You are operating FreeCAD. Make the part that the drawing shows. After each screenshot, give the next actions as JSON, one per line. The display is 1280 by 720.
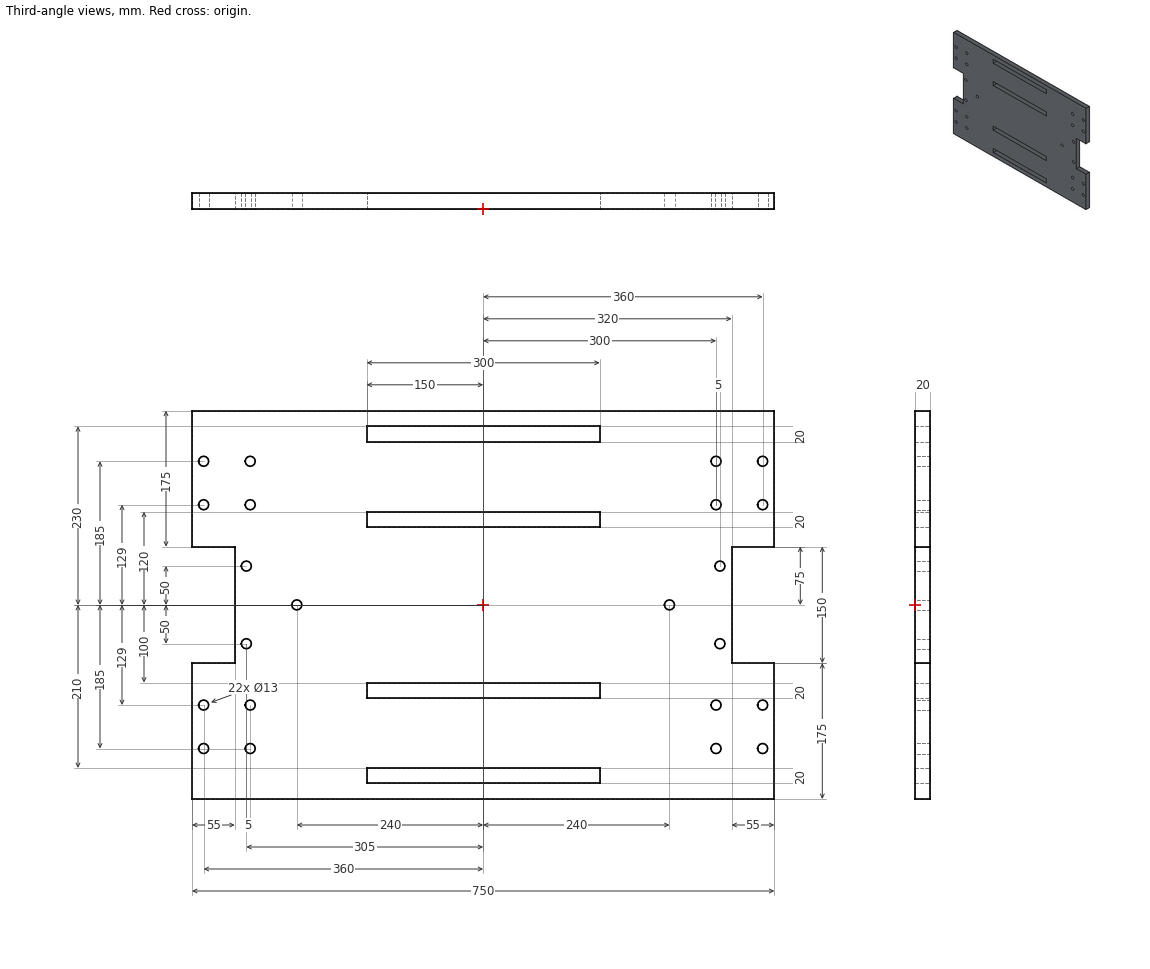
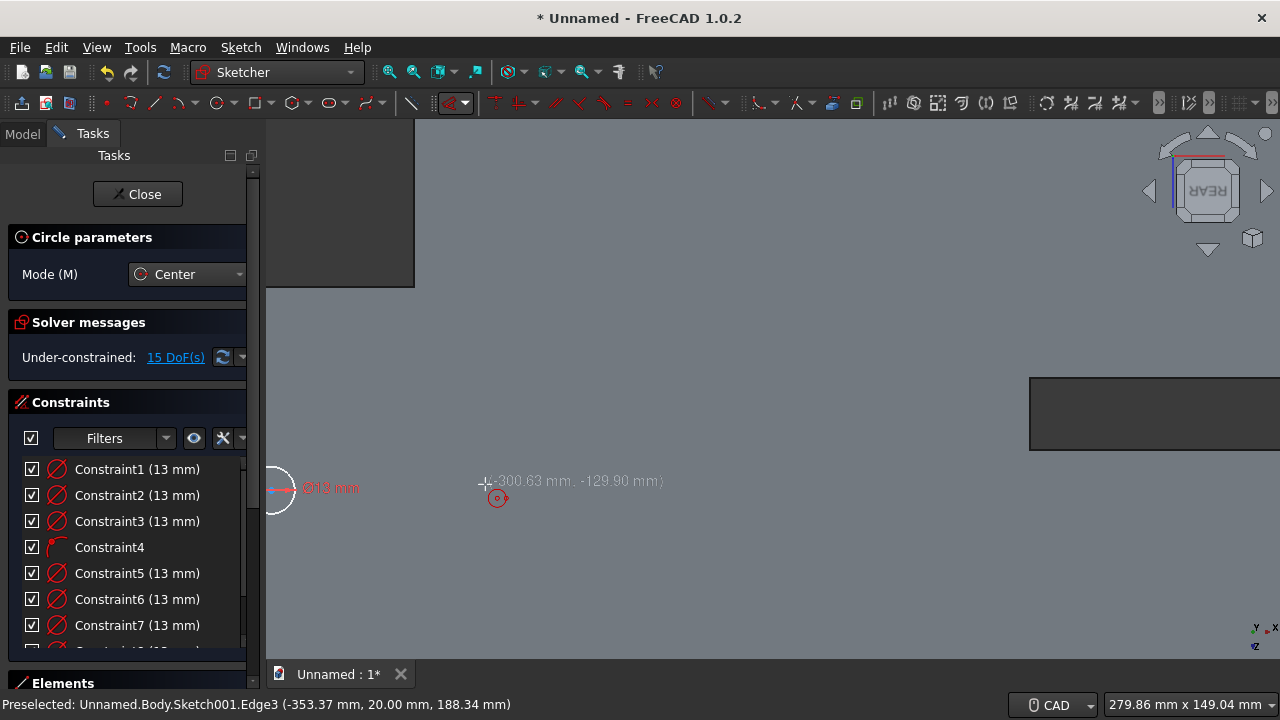
{"action": "scroll", "coordinate": [485, 483], "scroll_direction": "down", "scroll_amount": 8}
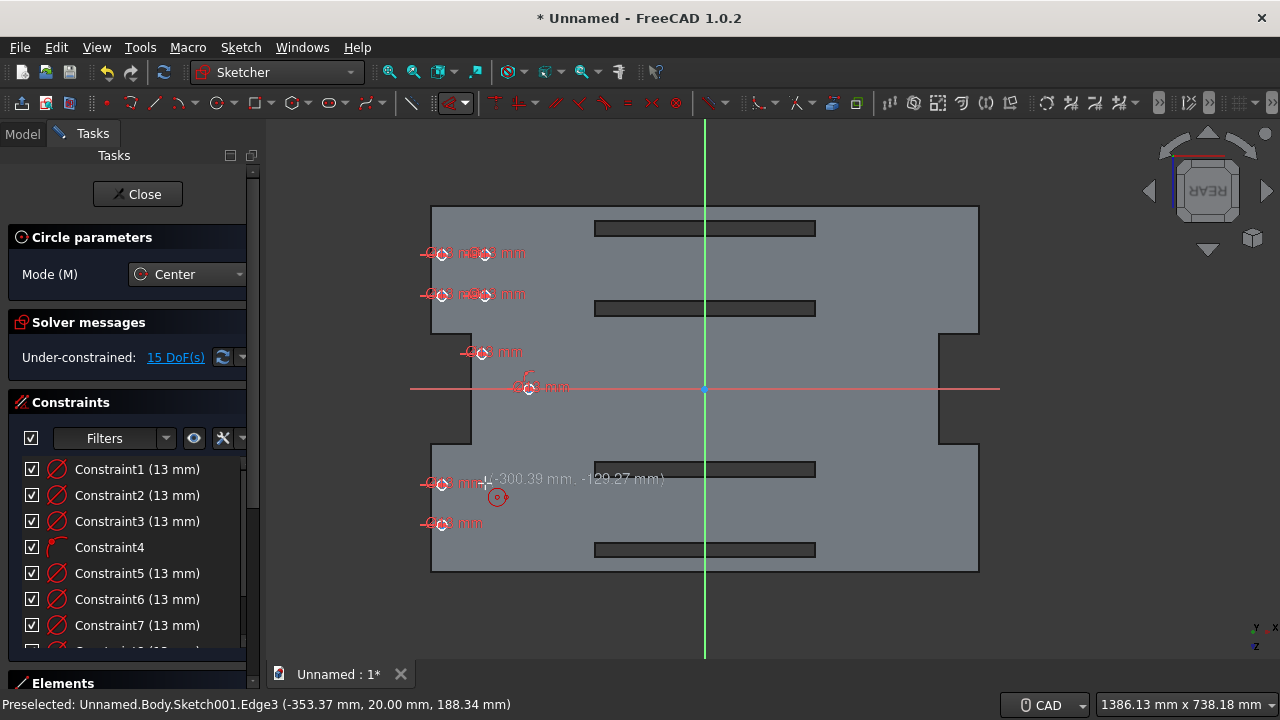
{"action": "left_click", "coordinate": [485, 484]}
{"action": "mouse_move", "coordinate": [489, 480]}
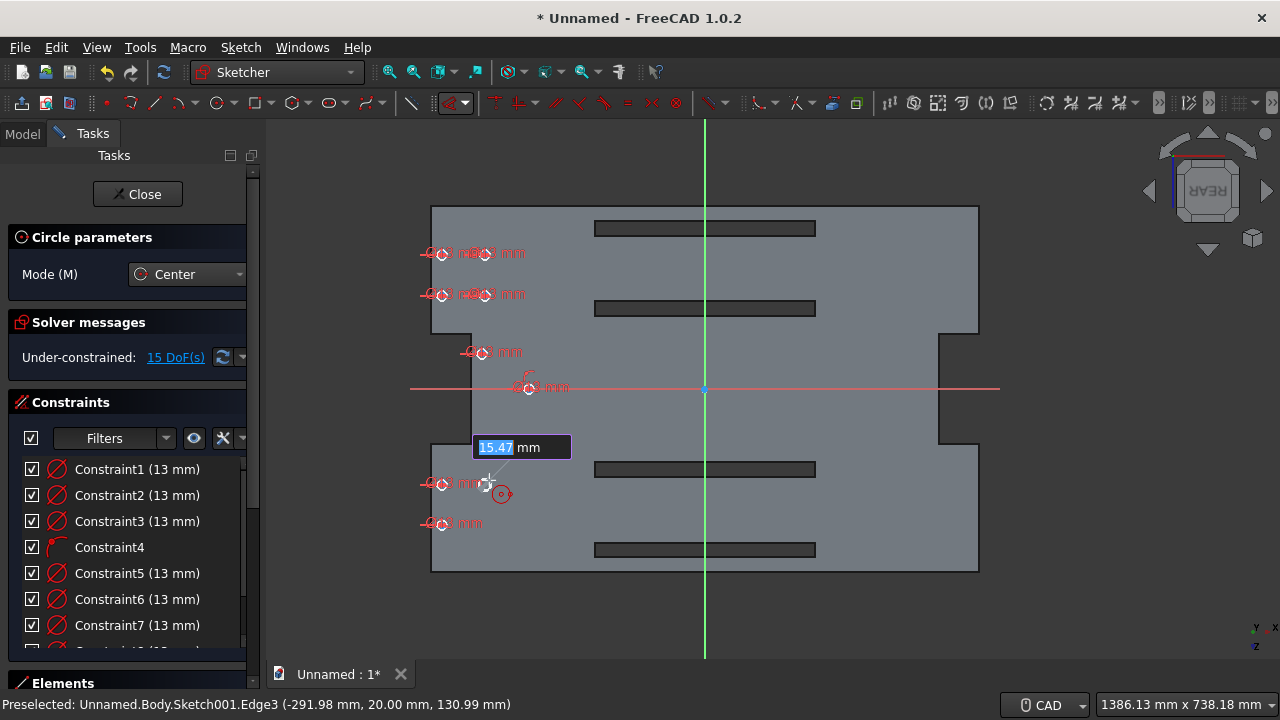
{"action": "type", "text": "13"}
{"action": "key", "text": "Return"}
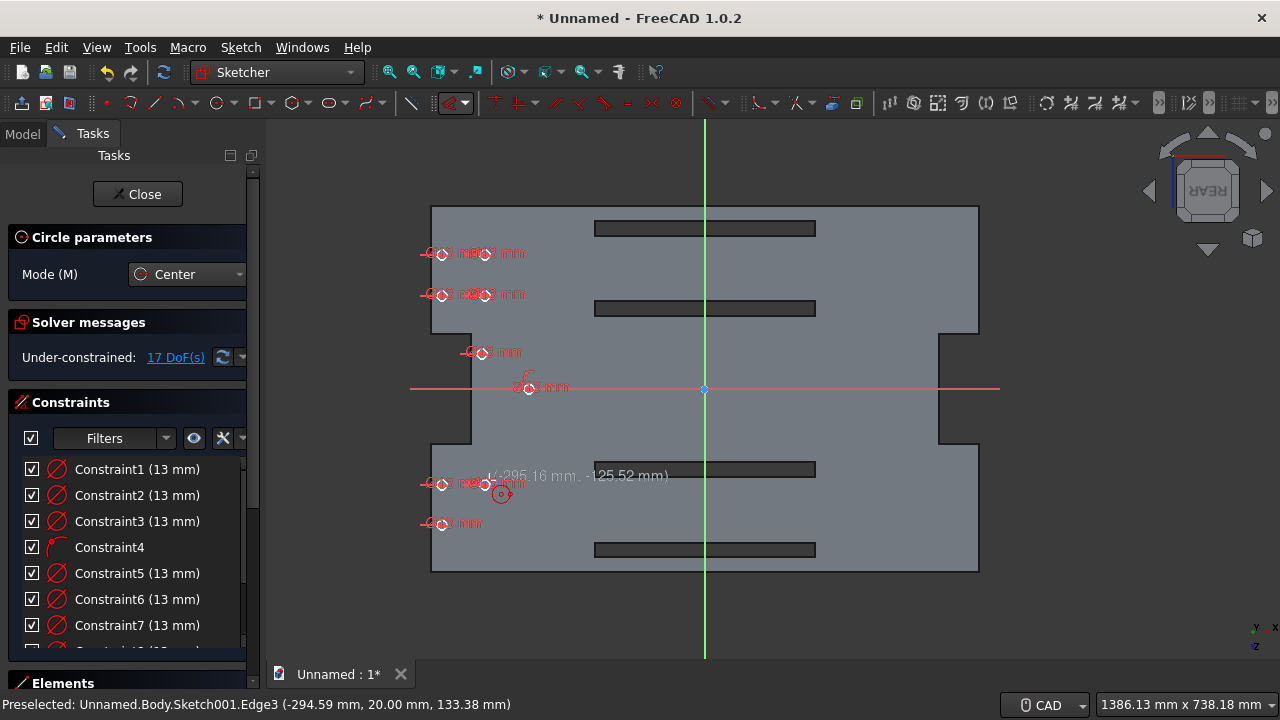
{"action": "scroll", "coordinate": [485, 525], "scroll_direction": "up", "scroll_amount": 8}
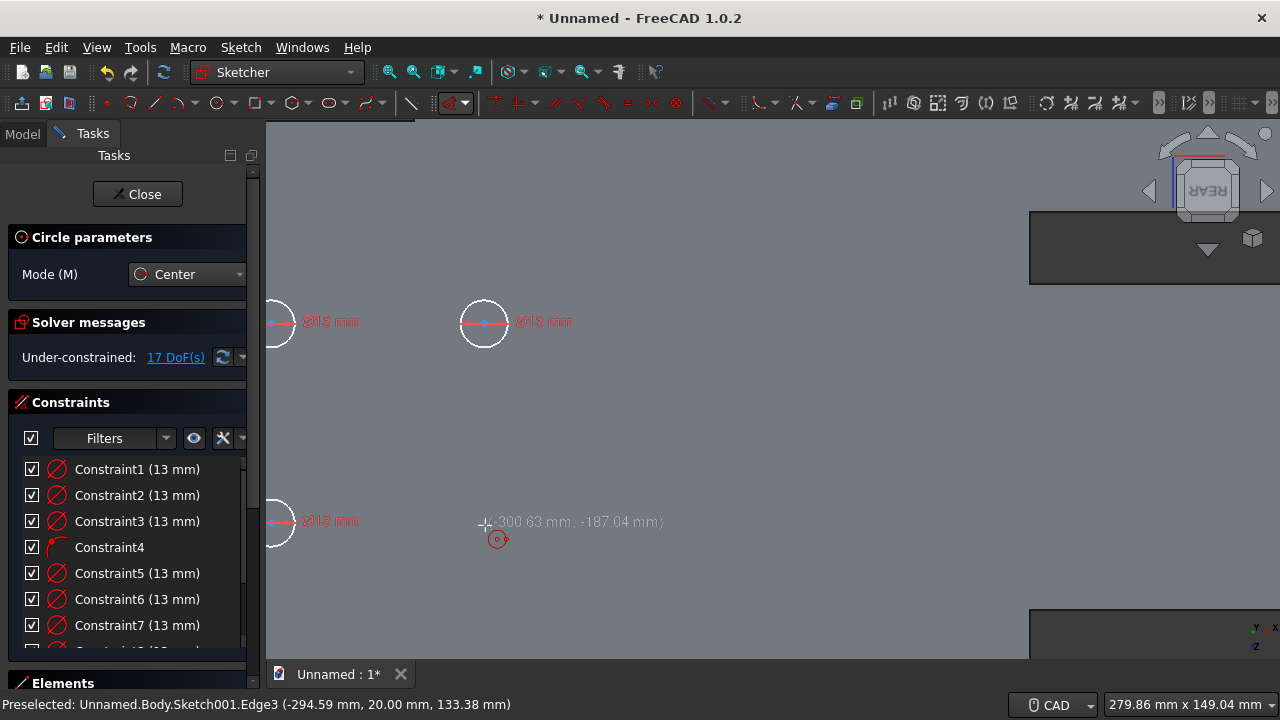
{"action": "scroll", "coordinate": [485, 526], "scroll_direction": "down", "scroll_amount": 8}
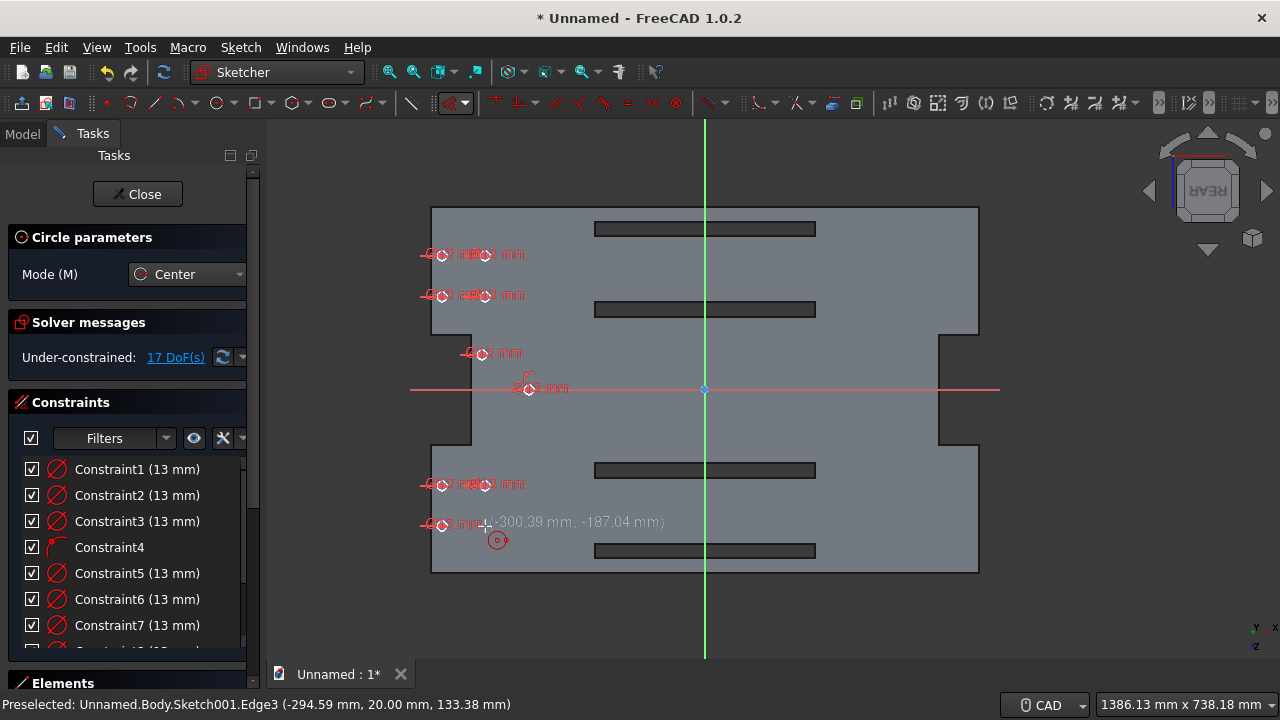
{"action": "left_click", "coordinate": [485, 525]}
{"action": "mouse_move", "coordinate": [489, 522]}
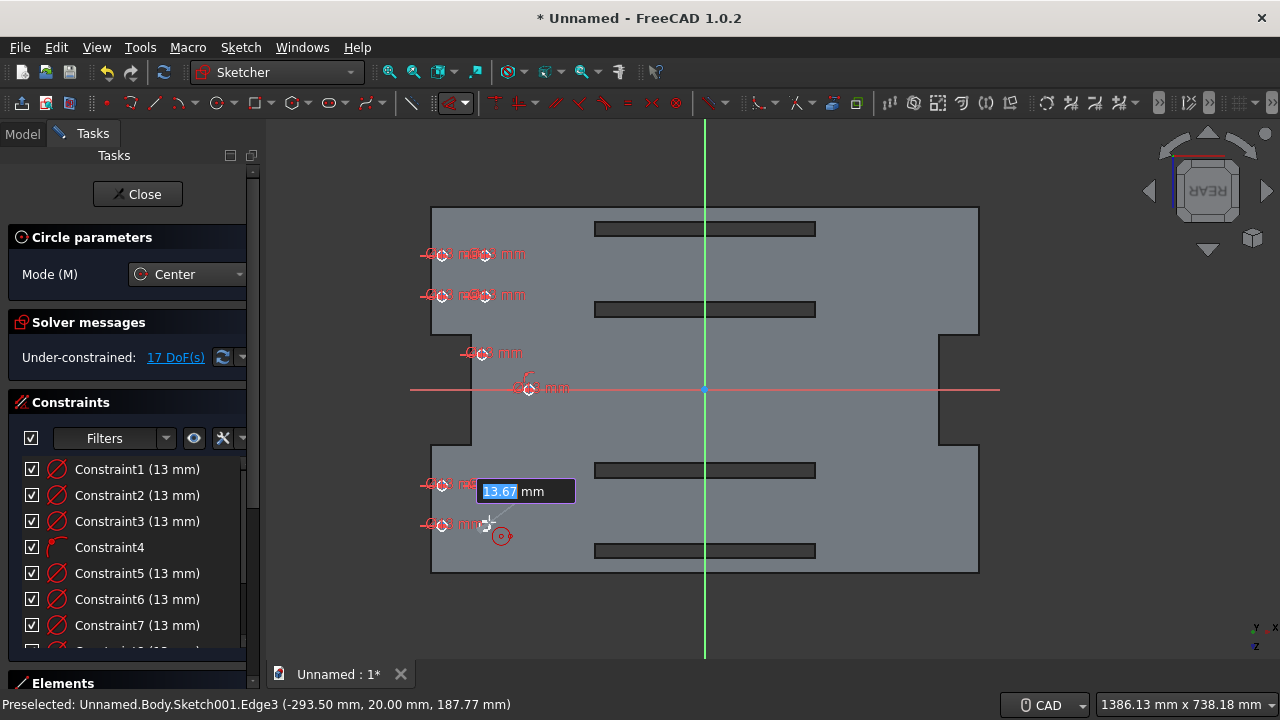
{"action": "type", "text": "13"}
{"action": "key", "text": "Return"}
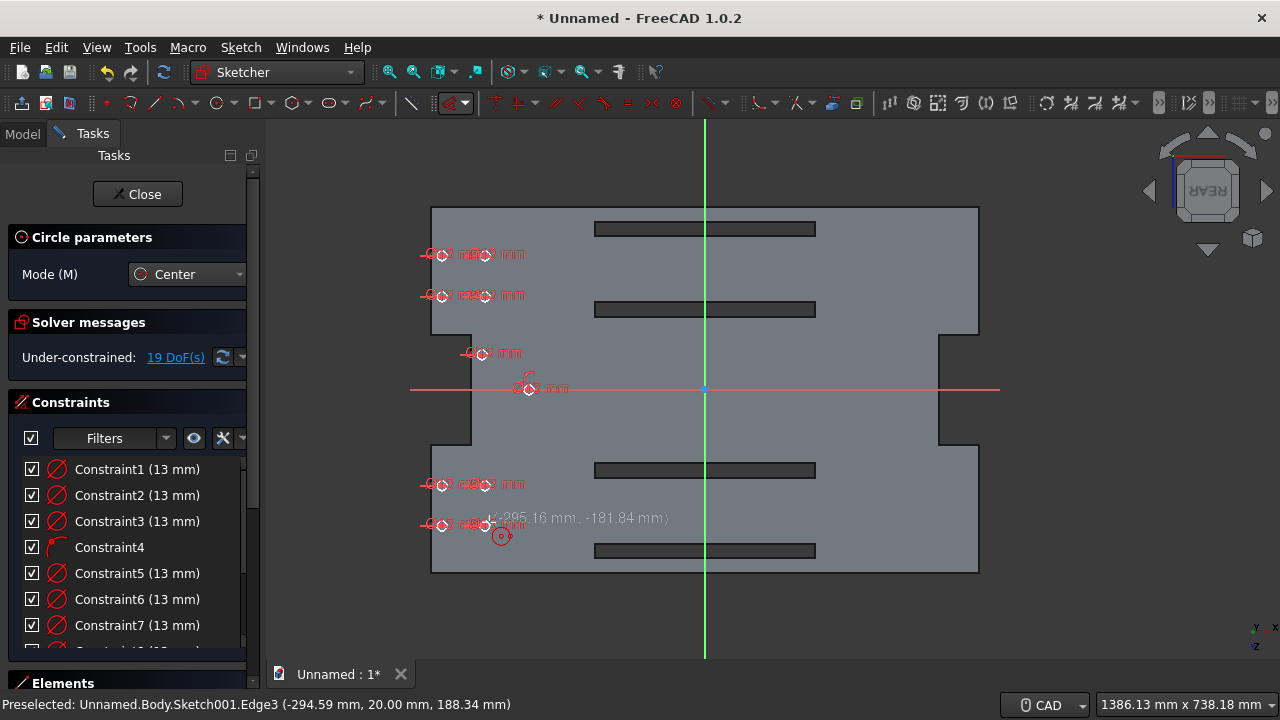
{"action": "scroll", "coordinate": [482, 427], "scroll_direction": "up", "scroll_amount": 8}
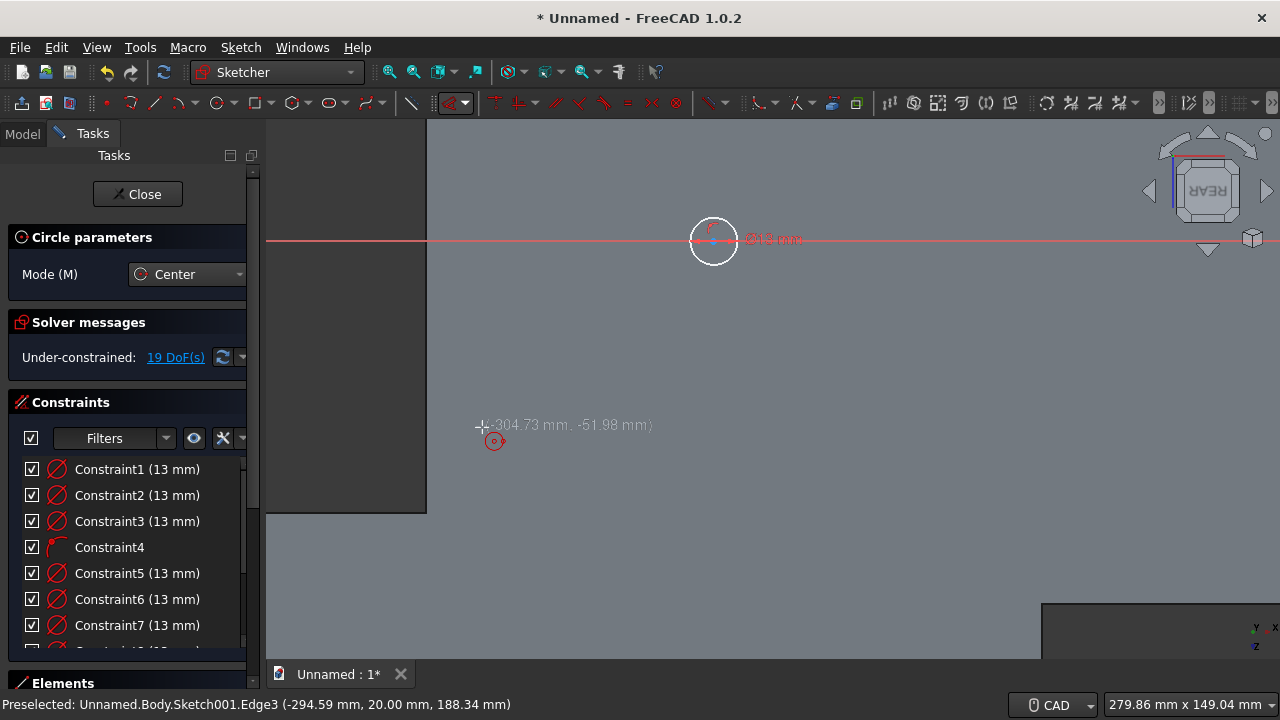
{"action": "scroll", "coordinate": [482, 426], "scroll_direction": "down", "scroll_amount": 8}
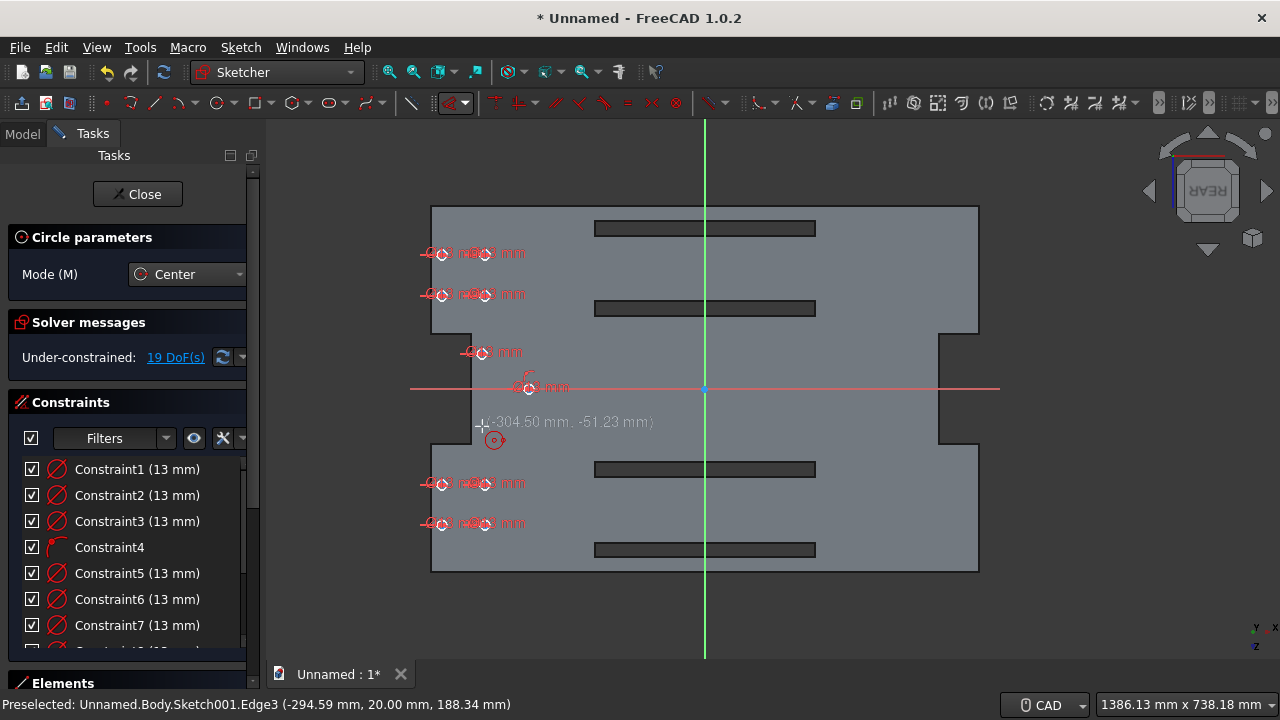
{"action": "left_click", "coordinate": [482, 426]}
{"action": "mouse_move", "coordinate": [485, 422]}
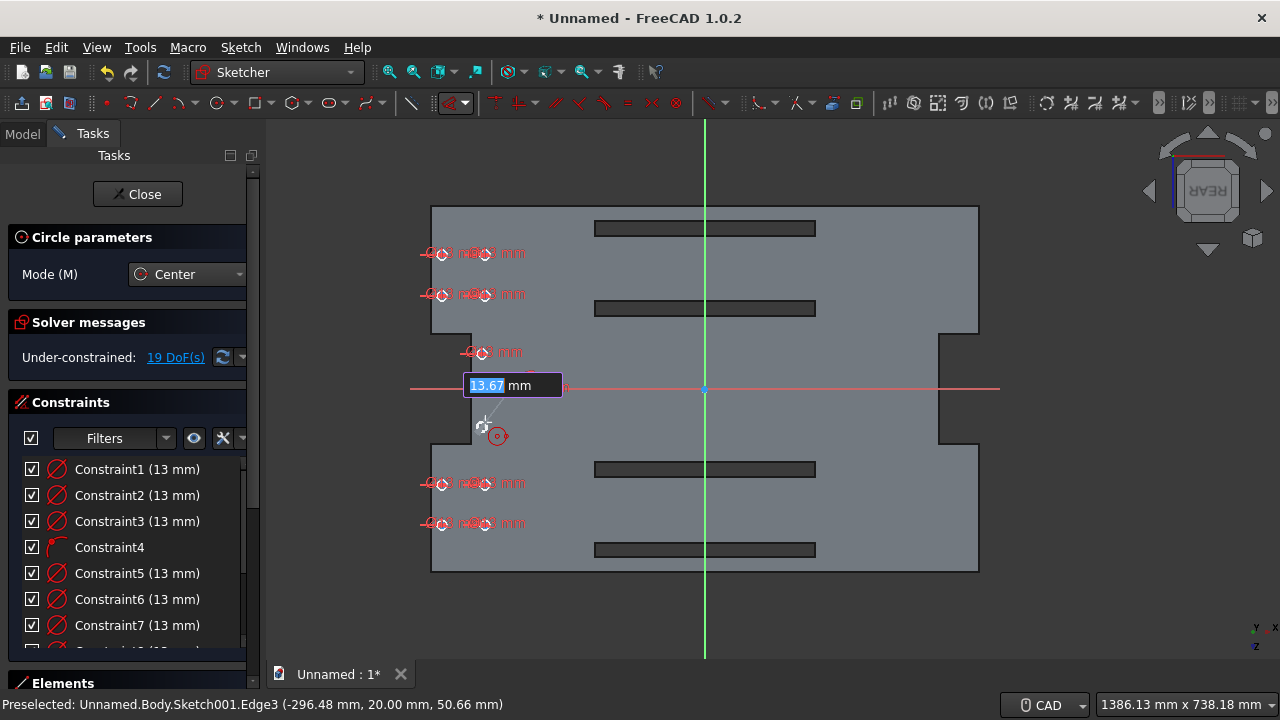
{"action": "type", "text": "13"}
{"action": "key", "text": "Return"}